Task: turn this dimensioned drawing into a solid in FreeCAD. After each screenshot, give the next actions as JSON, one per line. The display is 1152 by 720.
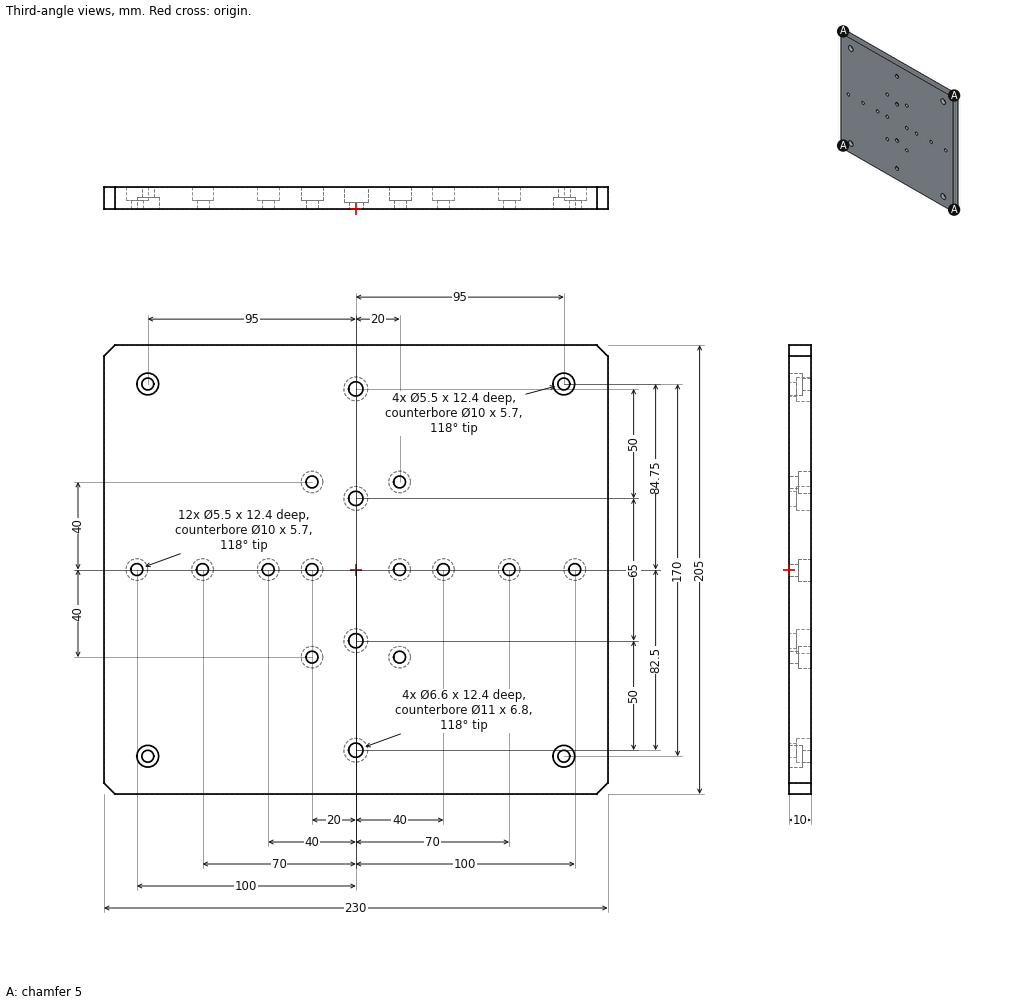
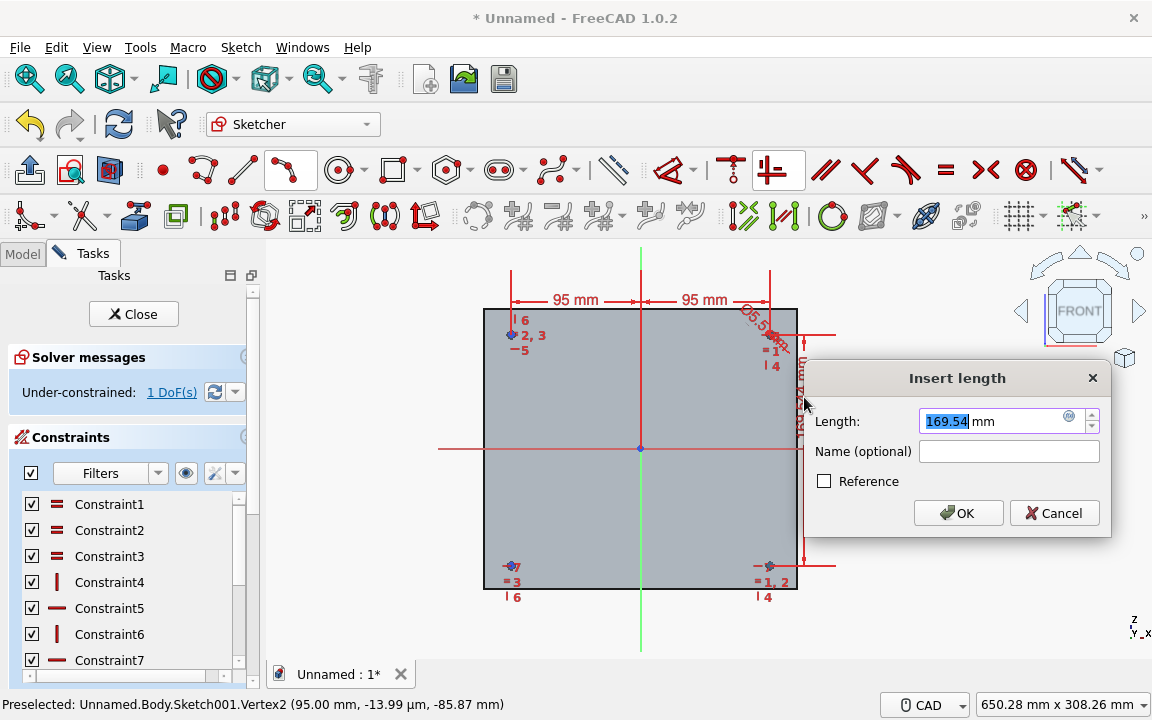
{"action": "type", "text": "170"}
{"action": "key", "text": "Return"}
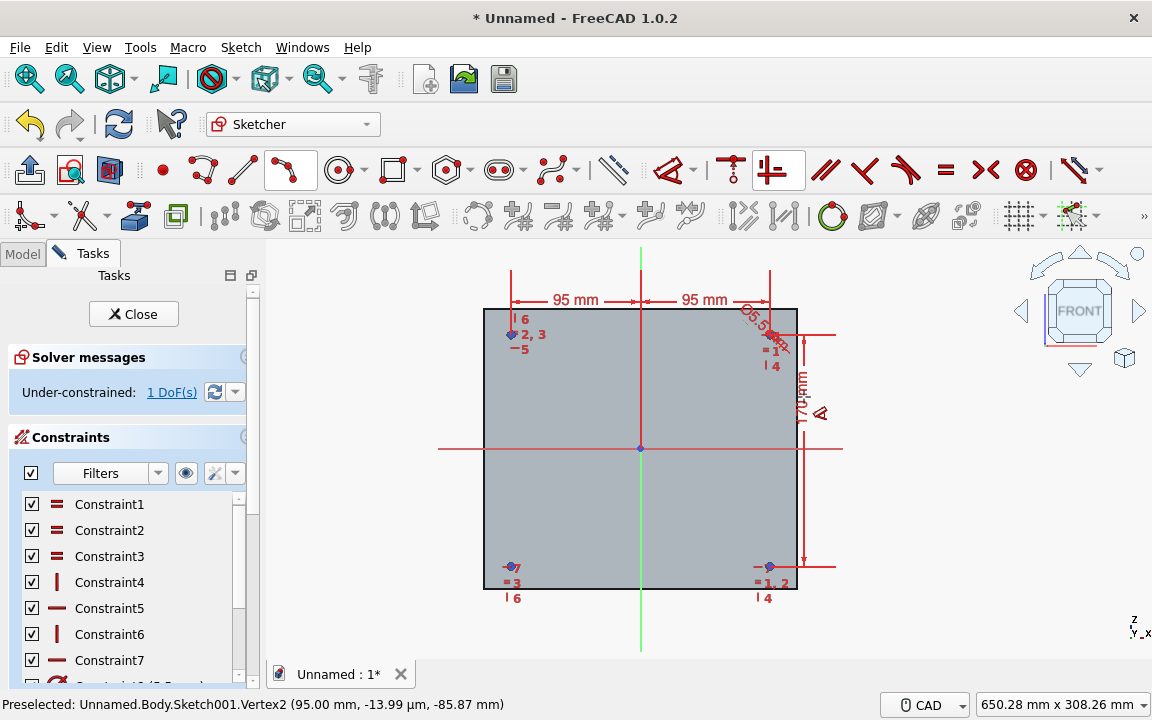
{"action": "left_click", "coordinate": [770, 335]}
{"action": "left_click", "coordinate": [804, 366]}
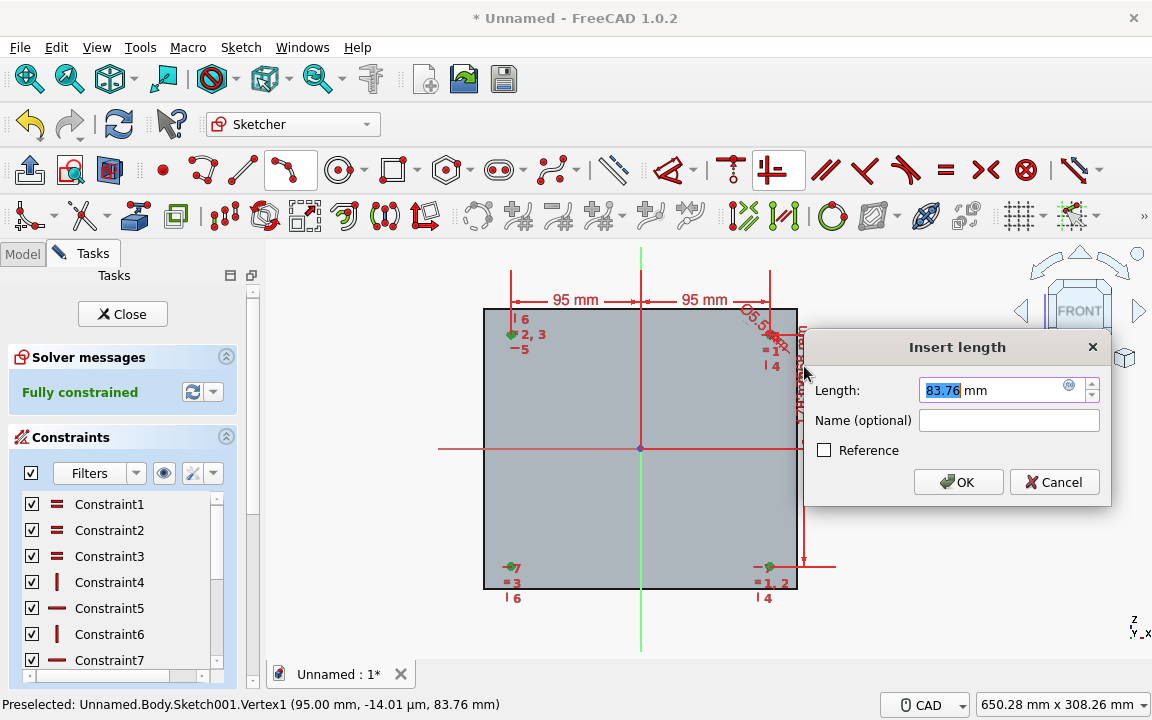
{"action": "type", "text": "84.75"}
{"action": "key", "text": "Return"}
{"action": "key", "text": "Escape"}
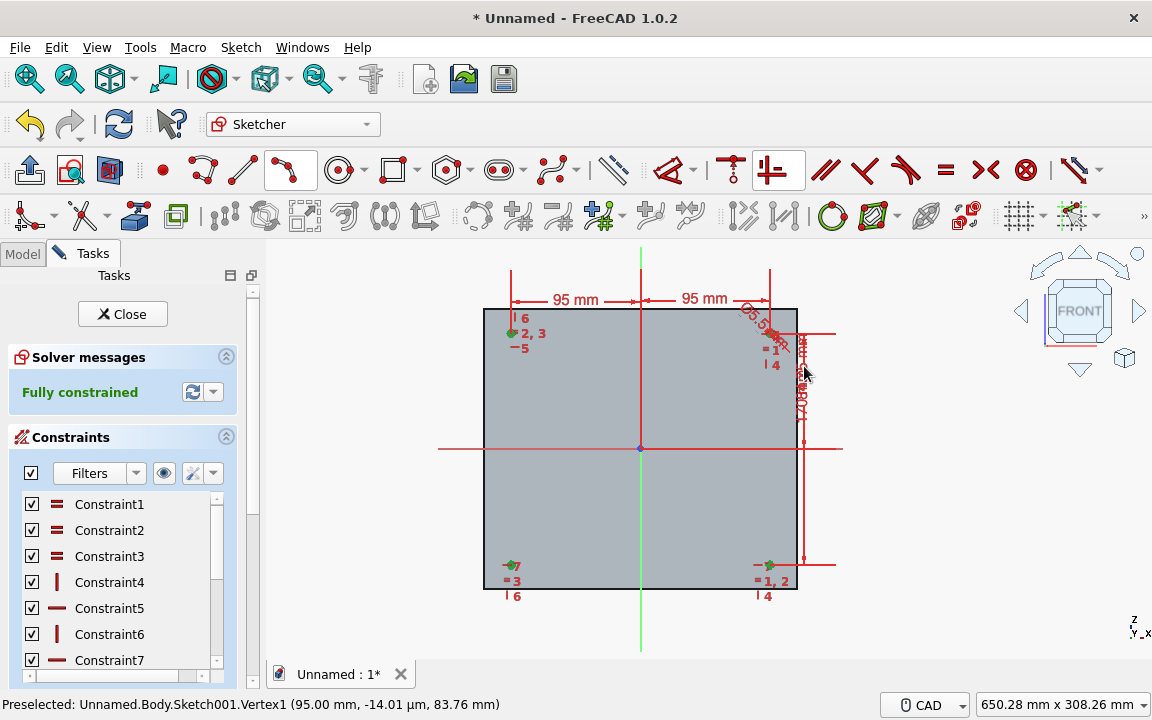
{"action": "left_click", "coordinate": [123, 314]}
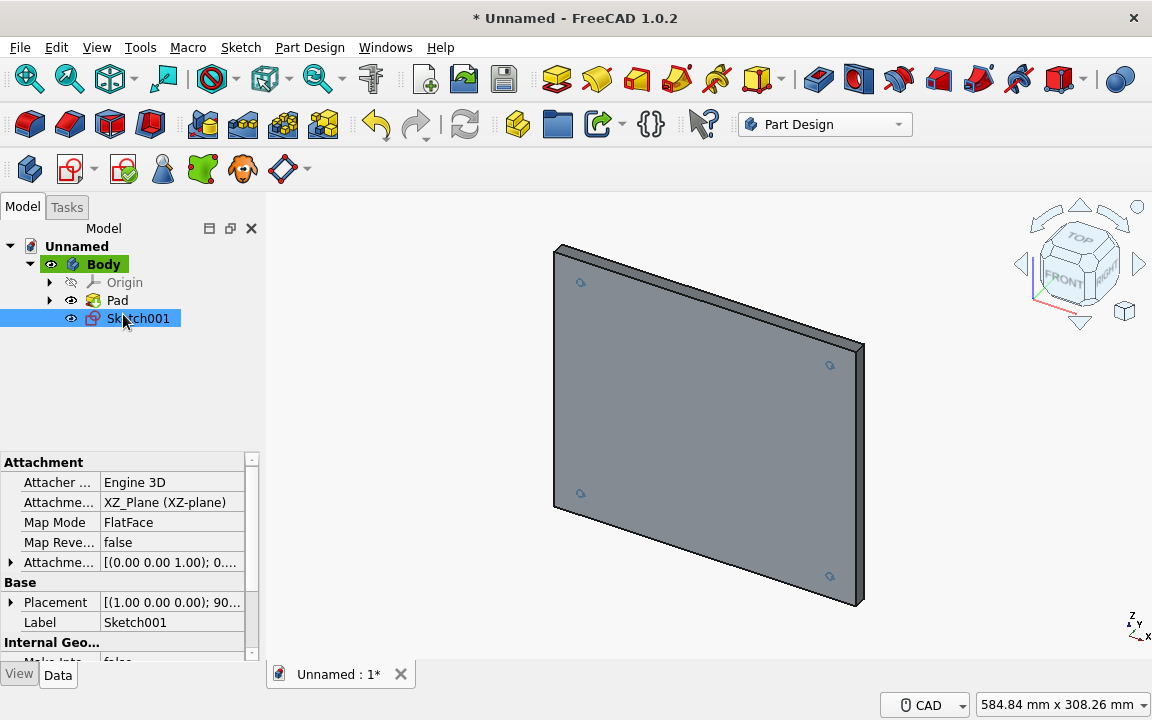
{"action": "left_click", "coordinate": [860, 80]}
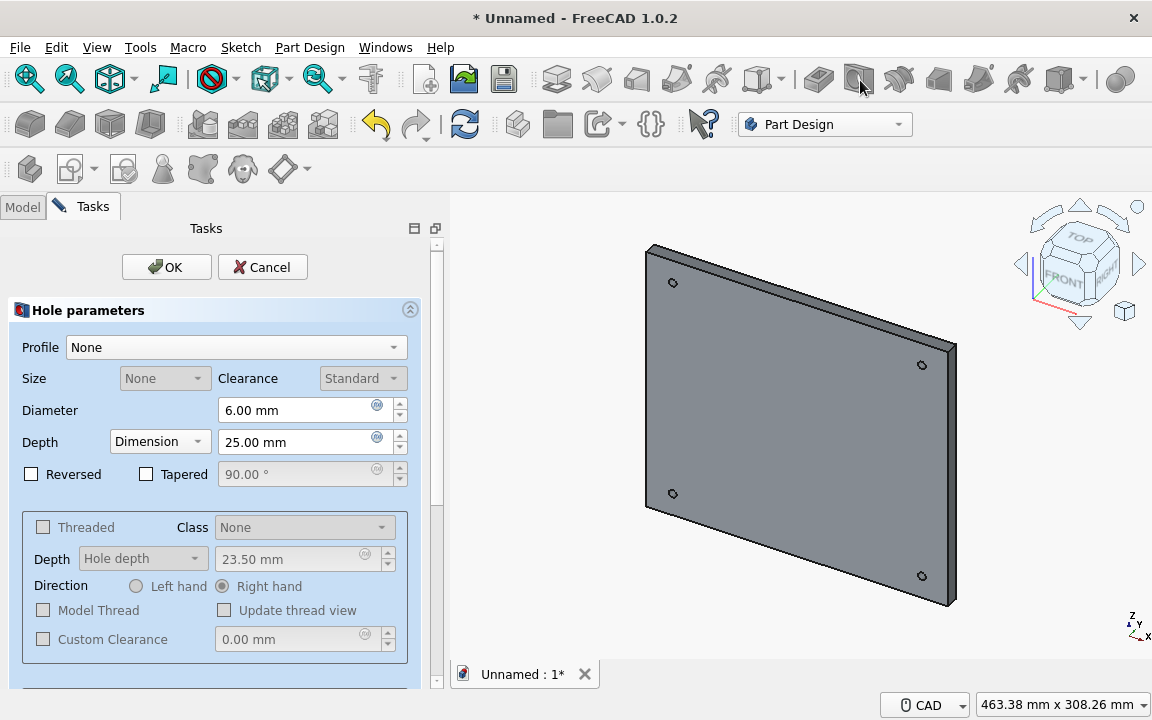
{"action": "triple_click", "coordinate": [305, 410]}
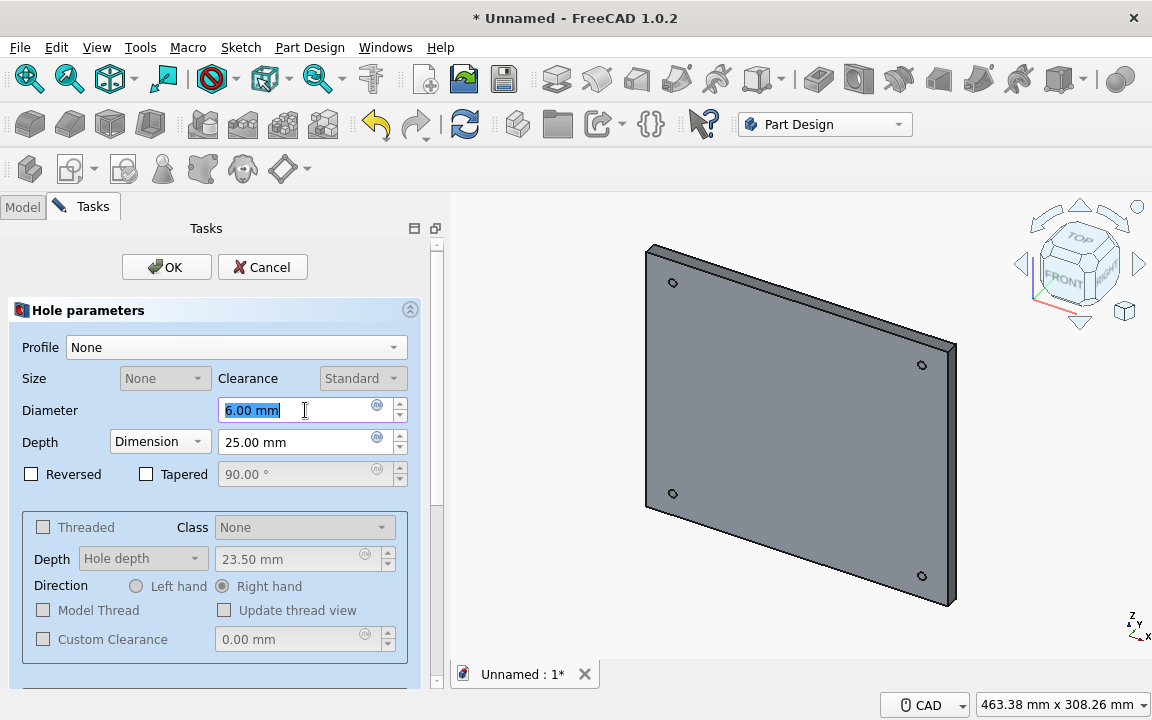
{"action": "type", "text": "5.5"}
{"action": "key", "text": "Tab"}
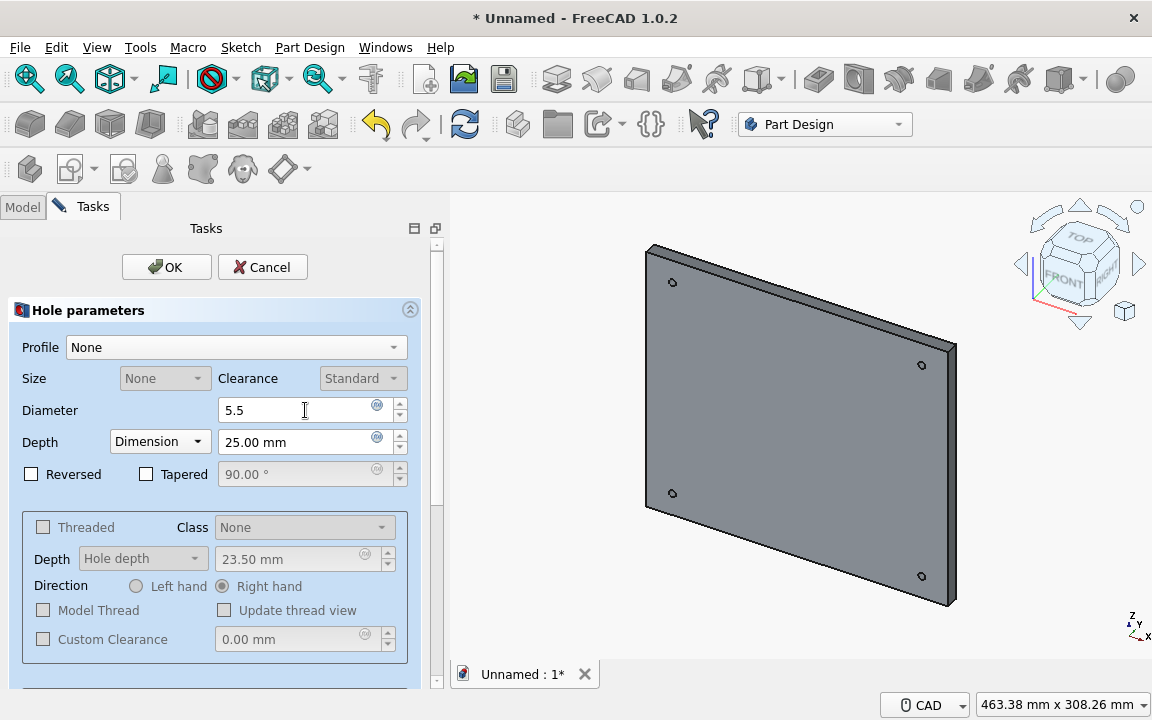
{"action": "triple_click", "coordinate": [305, 442]}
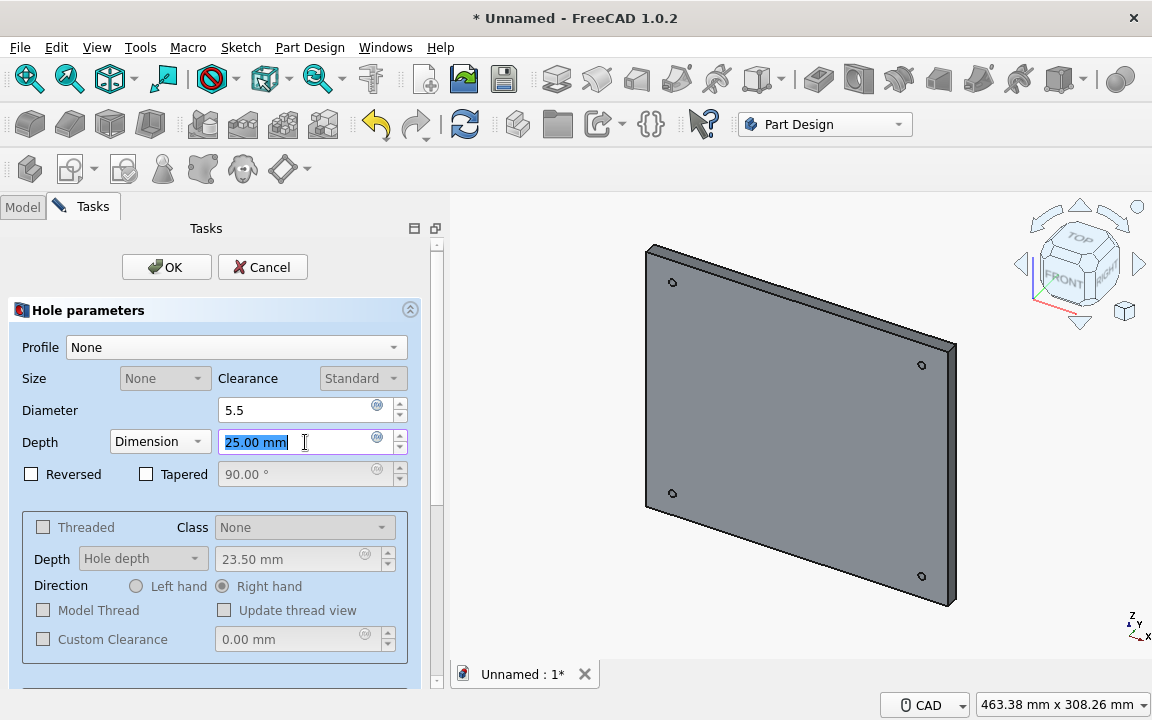
{"action": "type", "text": "12.4"}
{"action": "key", "text": "Tab"}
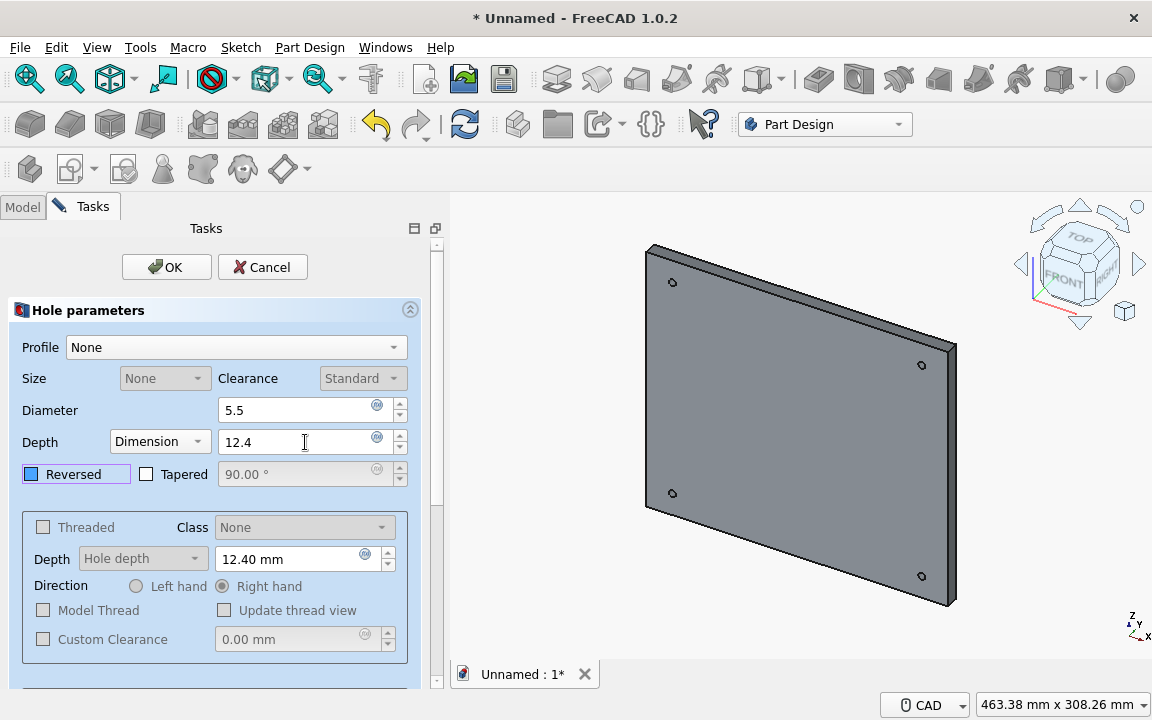
{"action": "scroll", "coordinate": [437, 463], "scroll_direction": "down", "scroll_amount": 2}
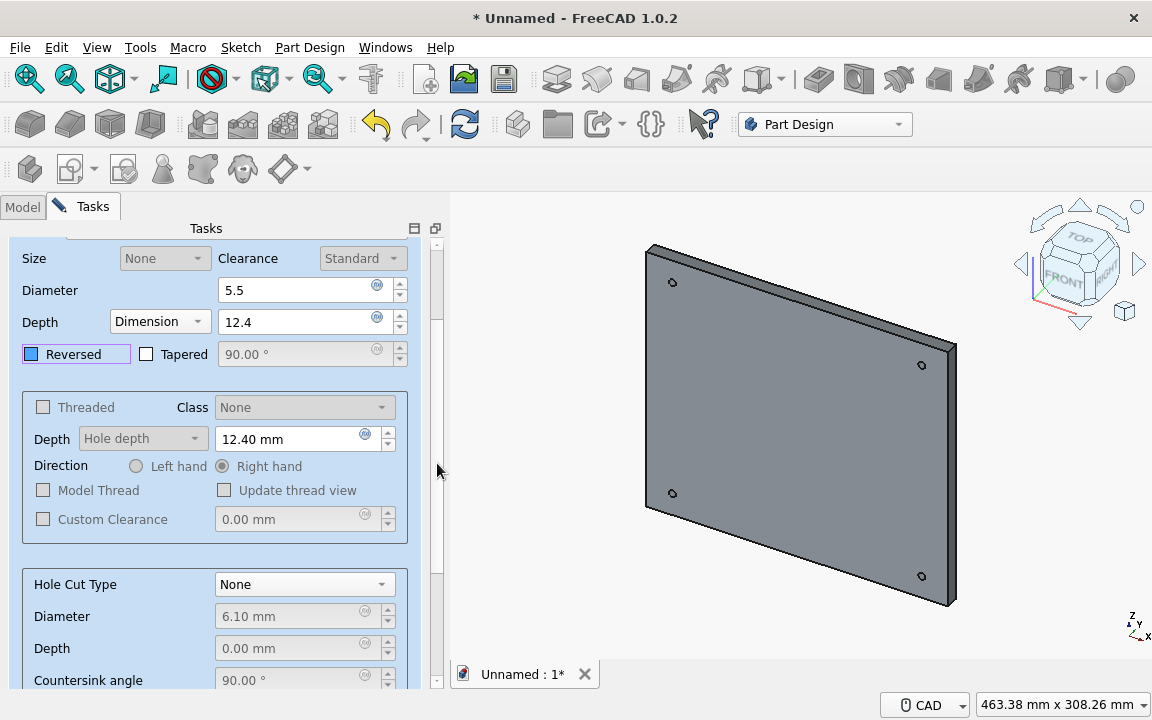
{"action": "left_click", "coordinate": [306, 584]}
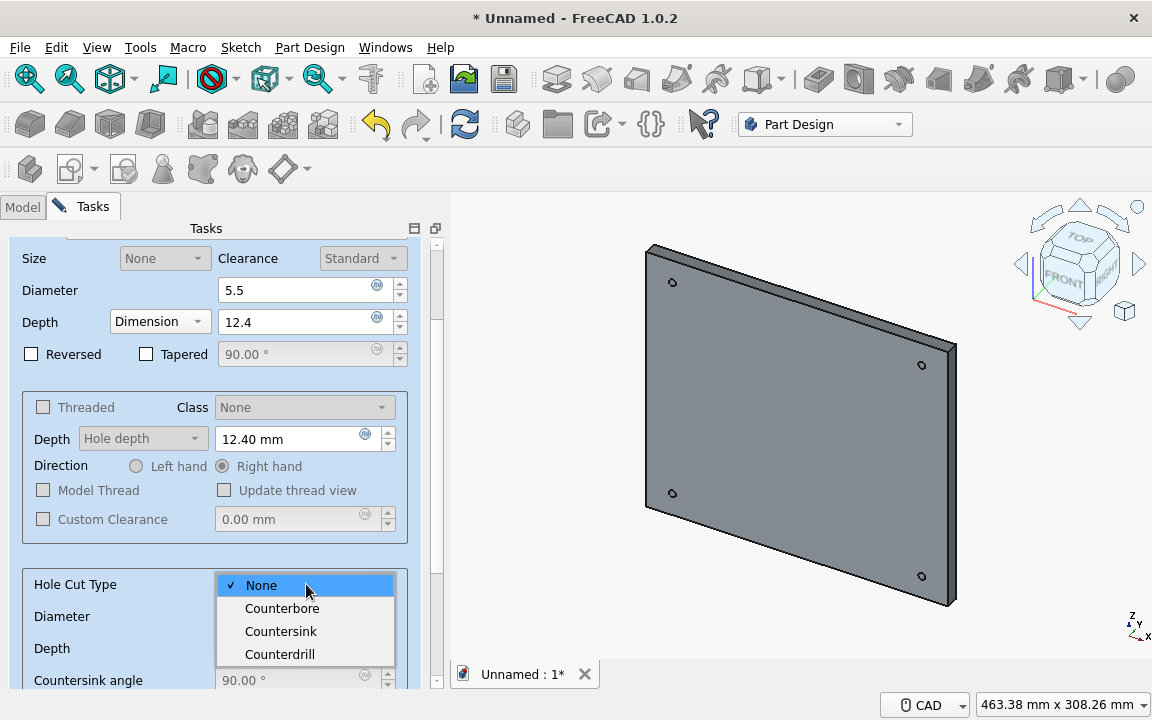
{"action": "left_click", "coordinate": [304, 608]}